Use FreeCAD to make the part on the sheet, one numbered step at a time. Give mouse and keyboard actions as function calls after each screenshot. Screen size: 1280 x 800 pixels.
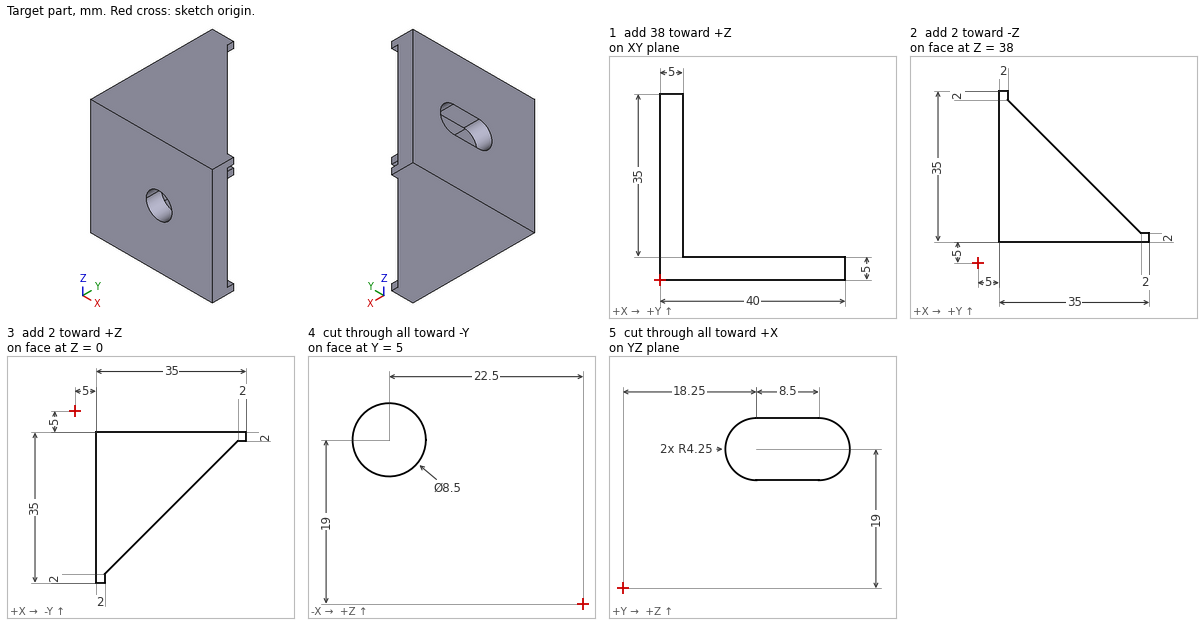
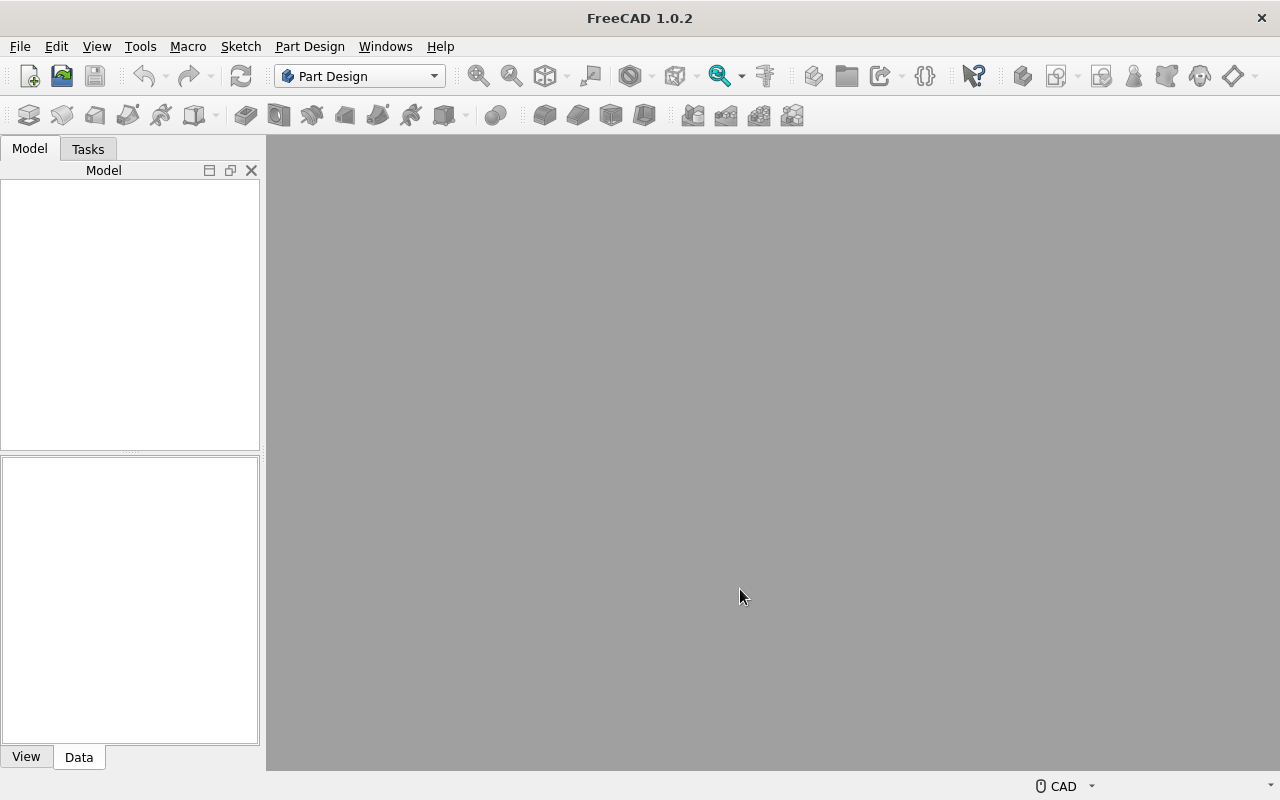
click(29, 76)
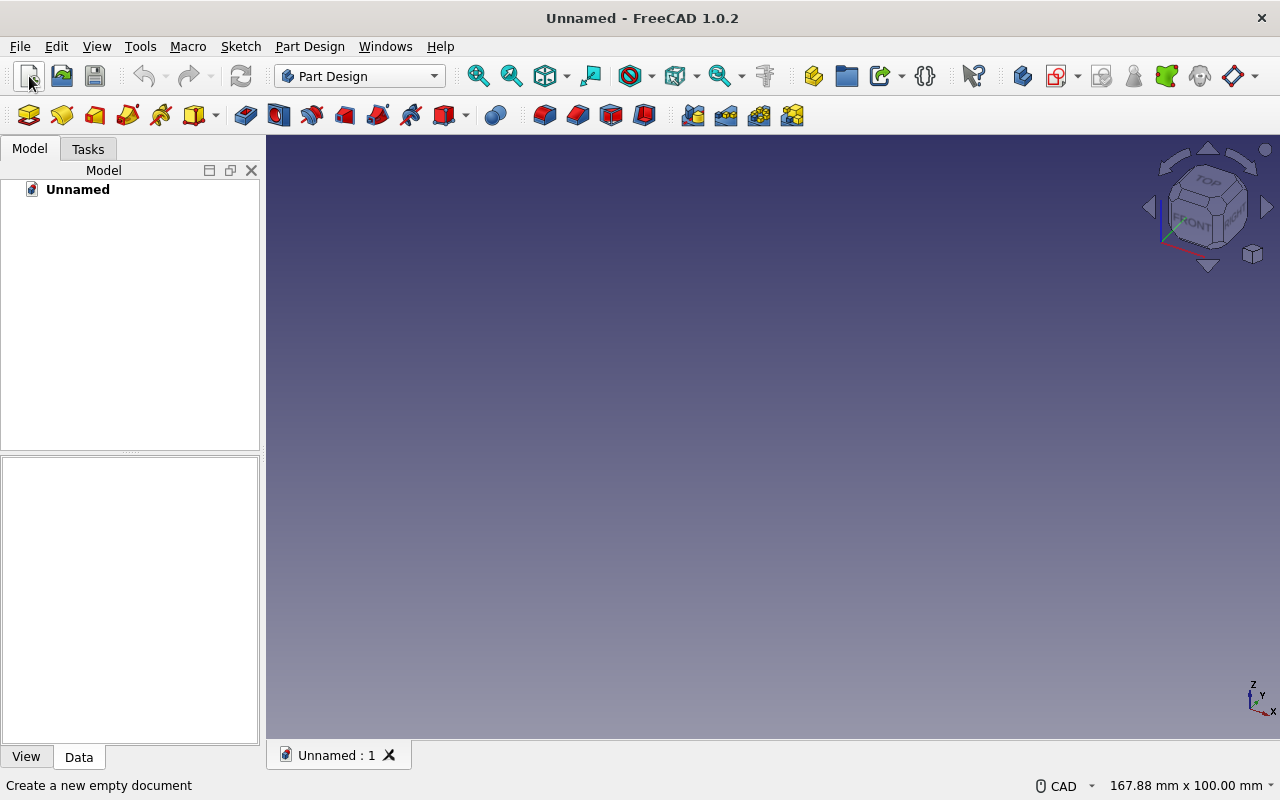
click(1056, 76)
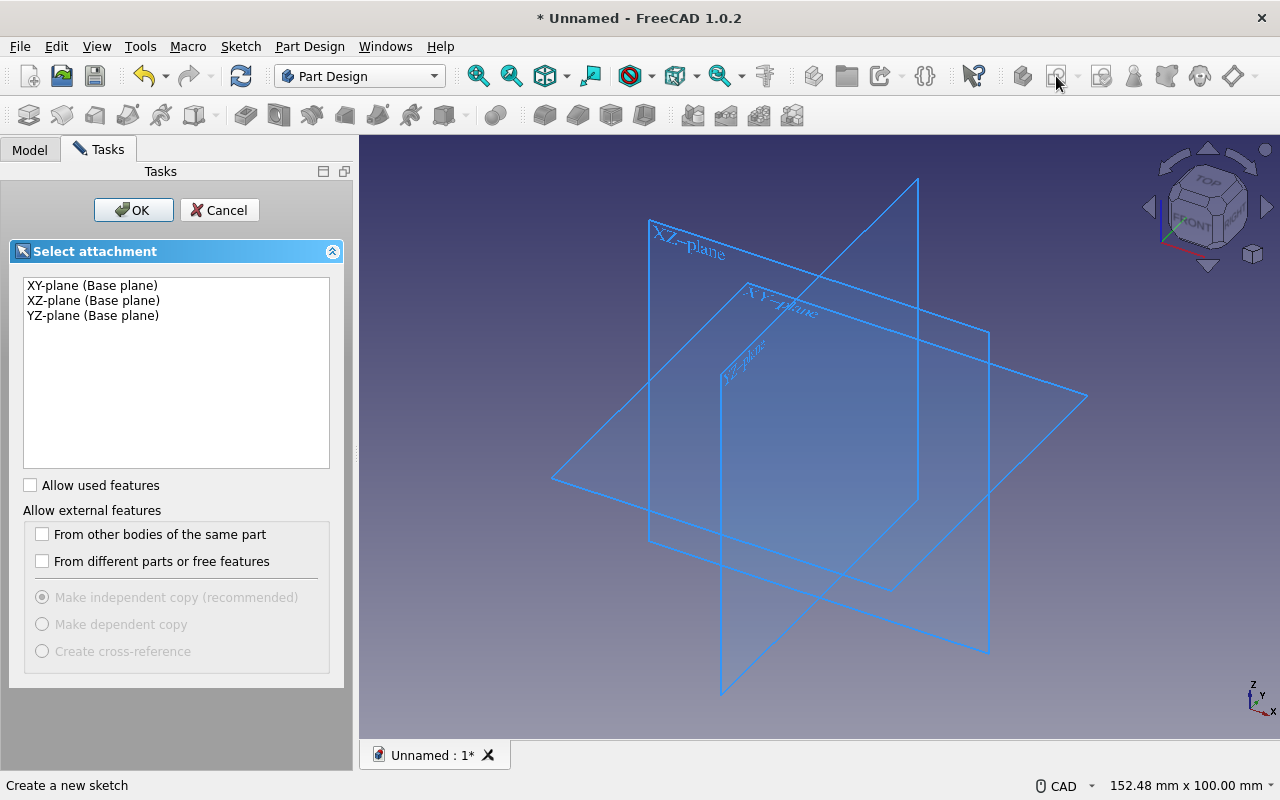
click(84, 286)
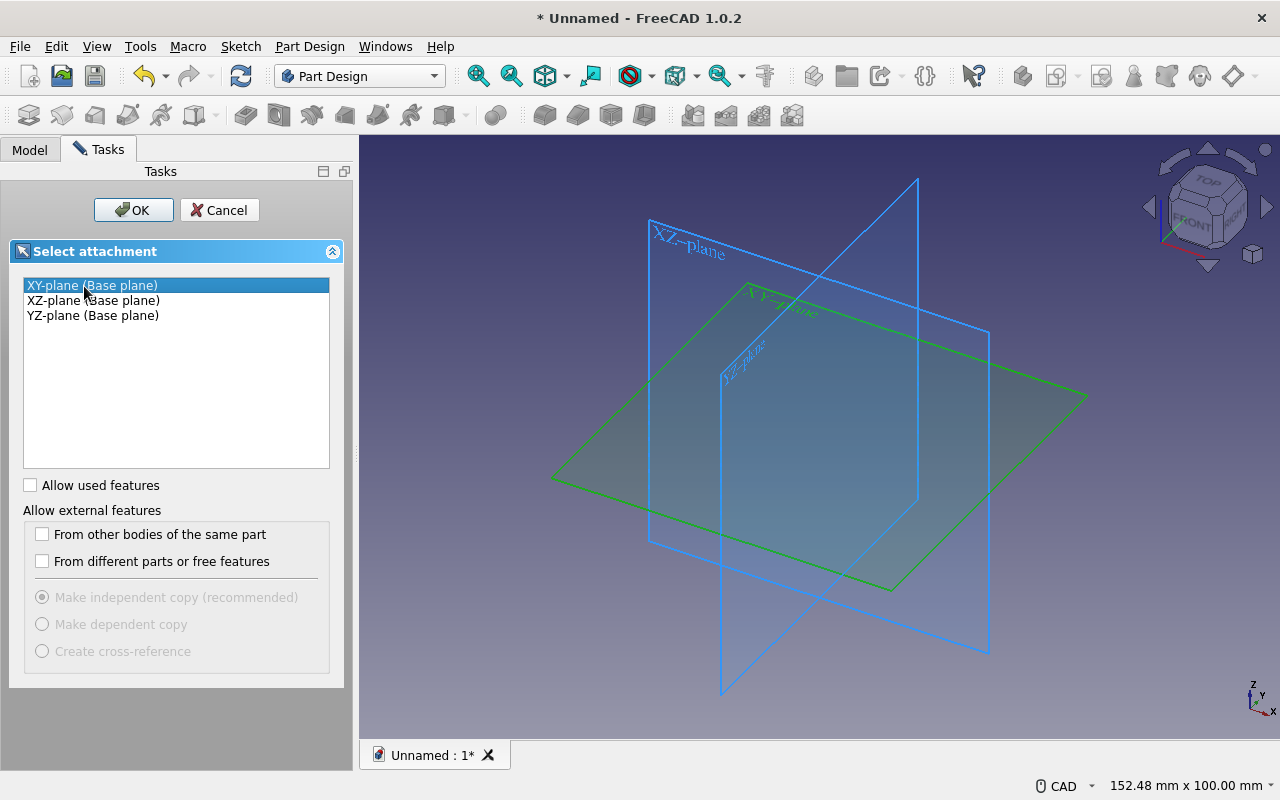
click(134, 210)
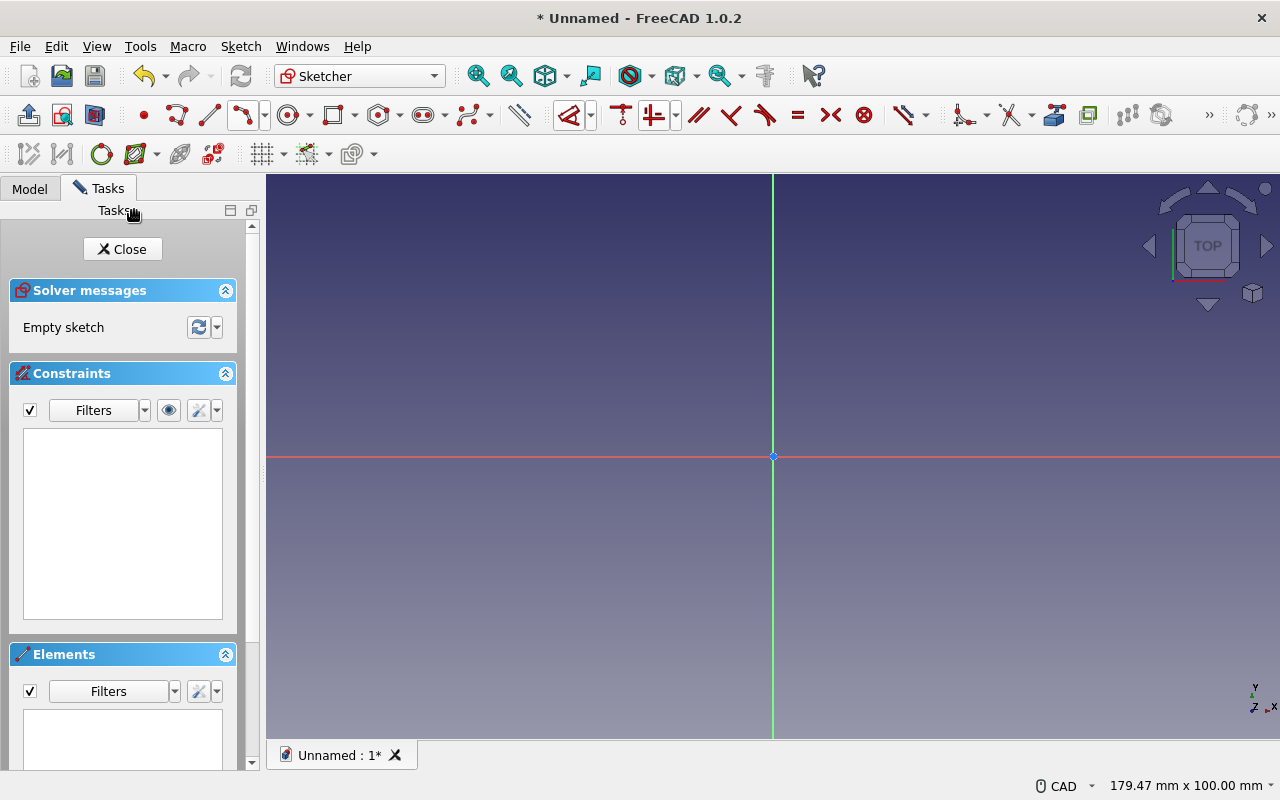
scroll(1115, 202, up, 2)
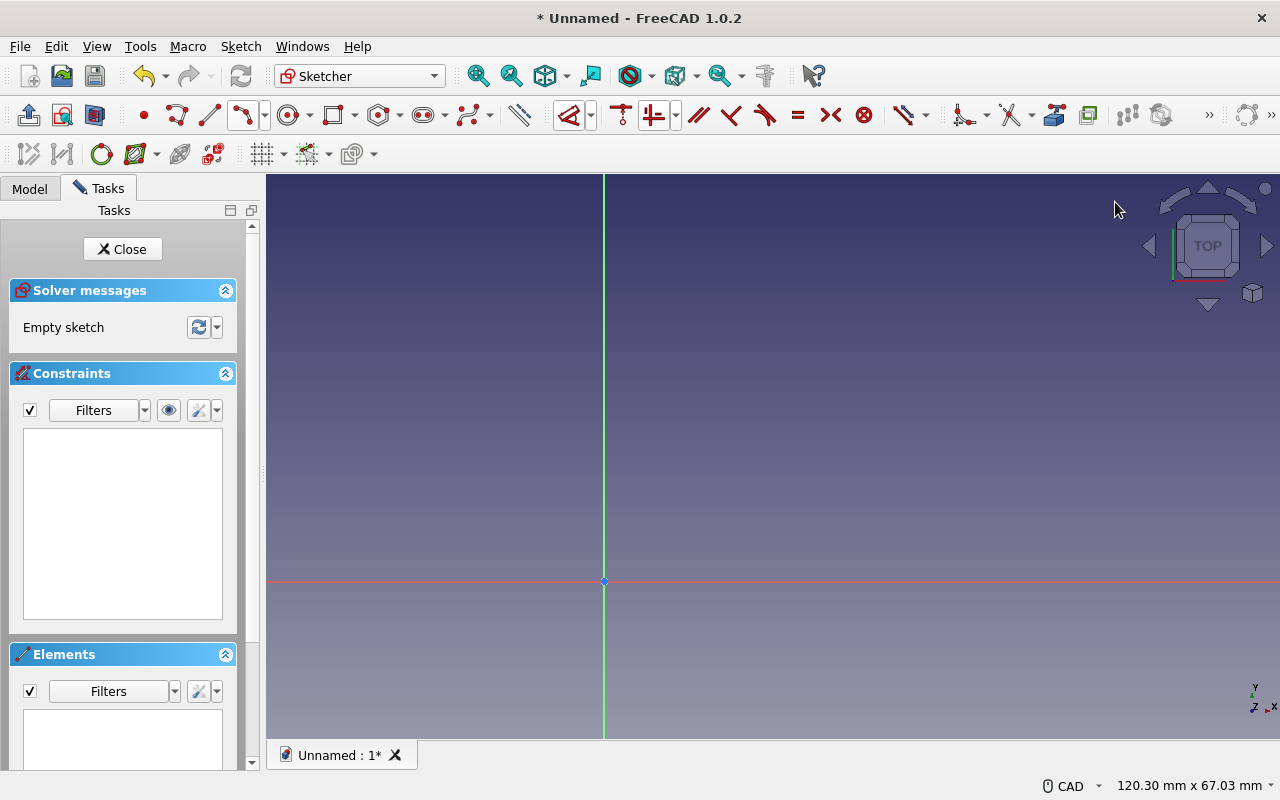
click(177, 116)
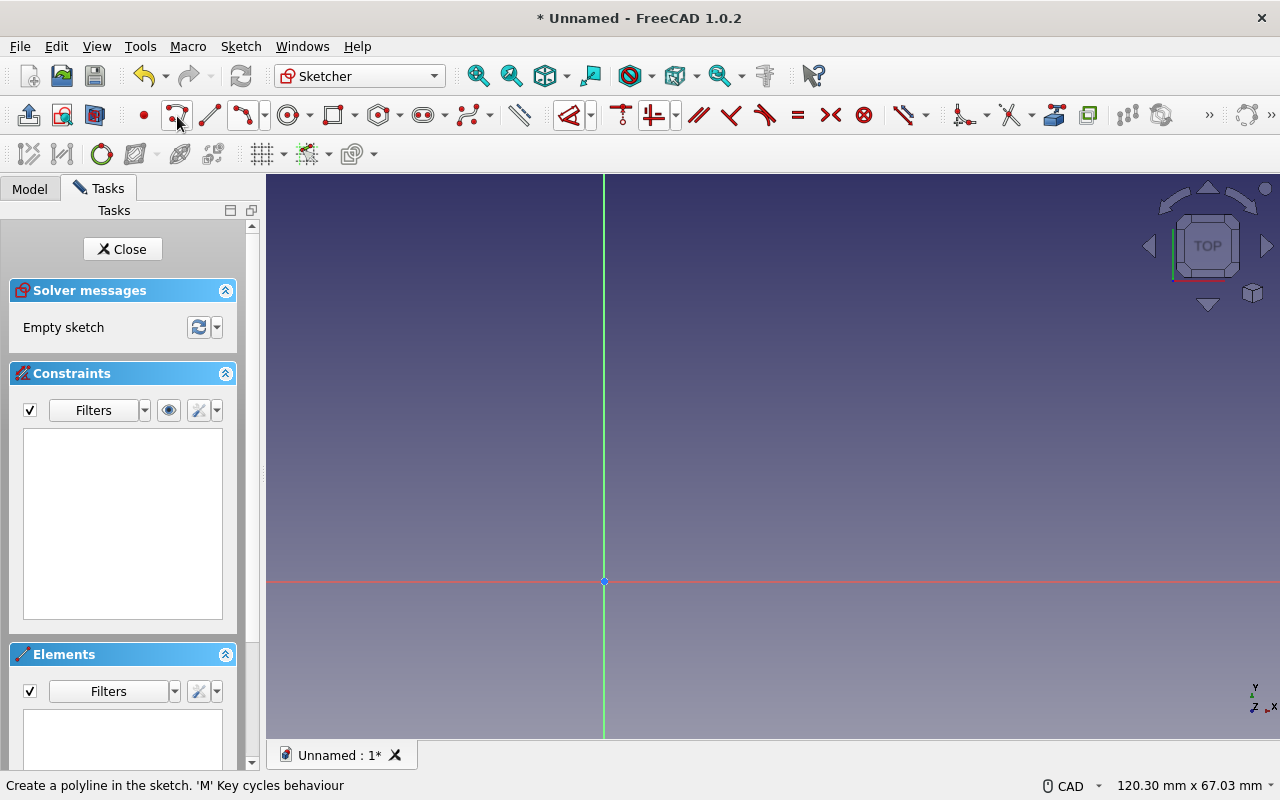
click(604, 582)
click(942, 573)
click(942, 540)
click(647, 540)
click(647, 244)
click(613, 244)
click(604, 582)
key(Escape)
key(Escape)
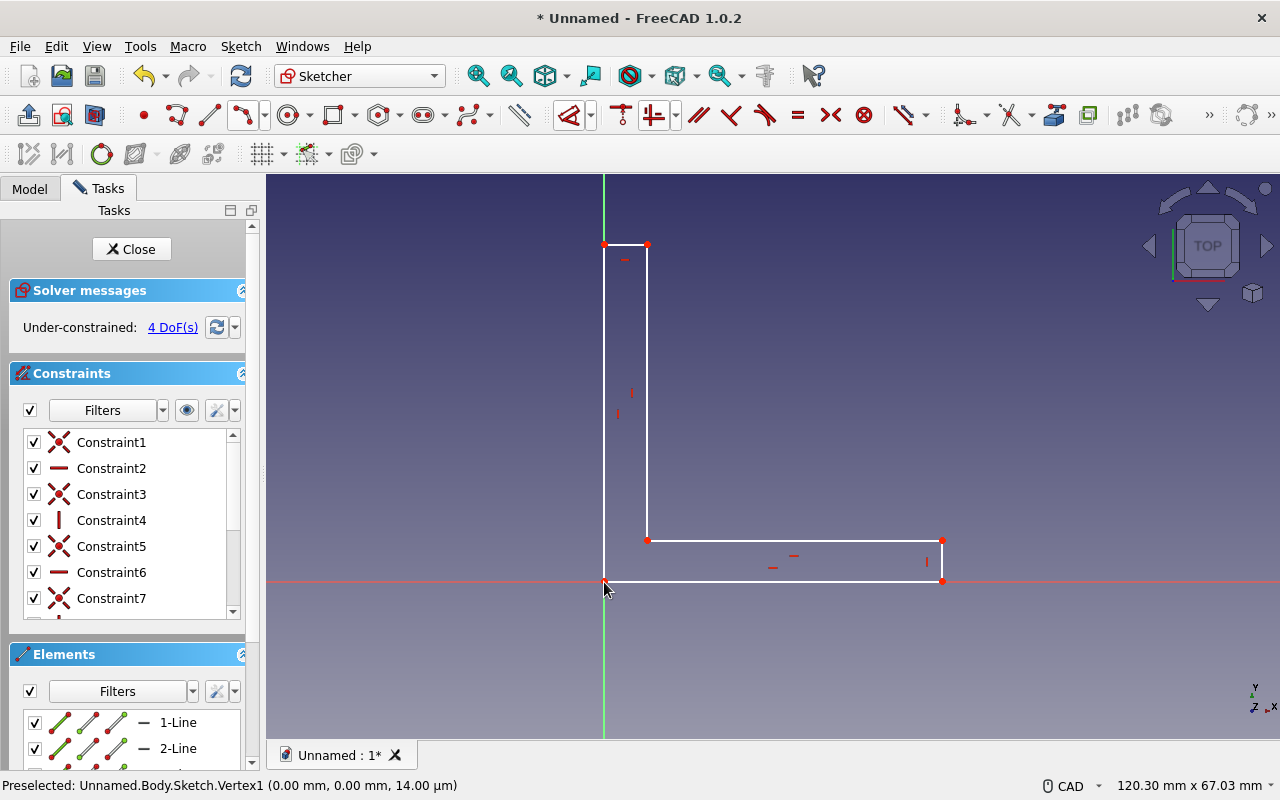
click(942, 569)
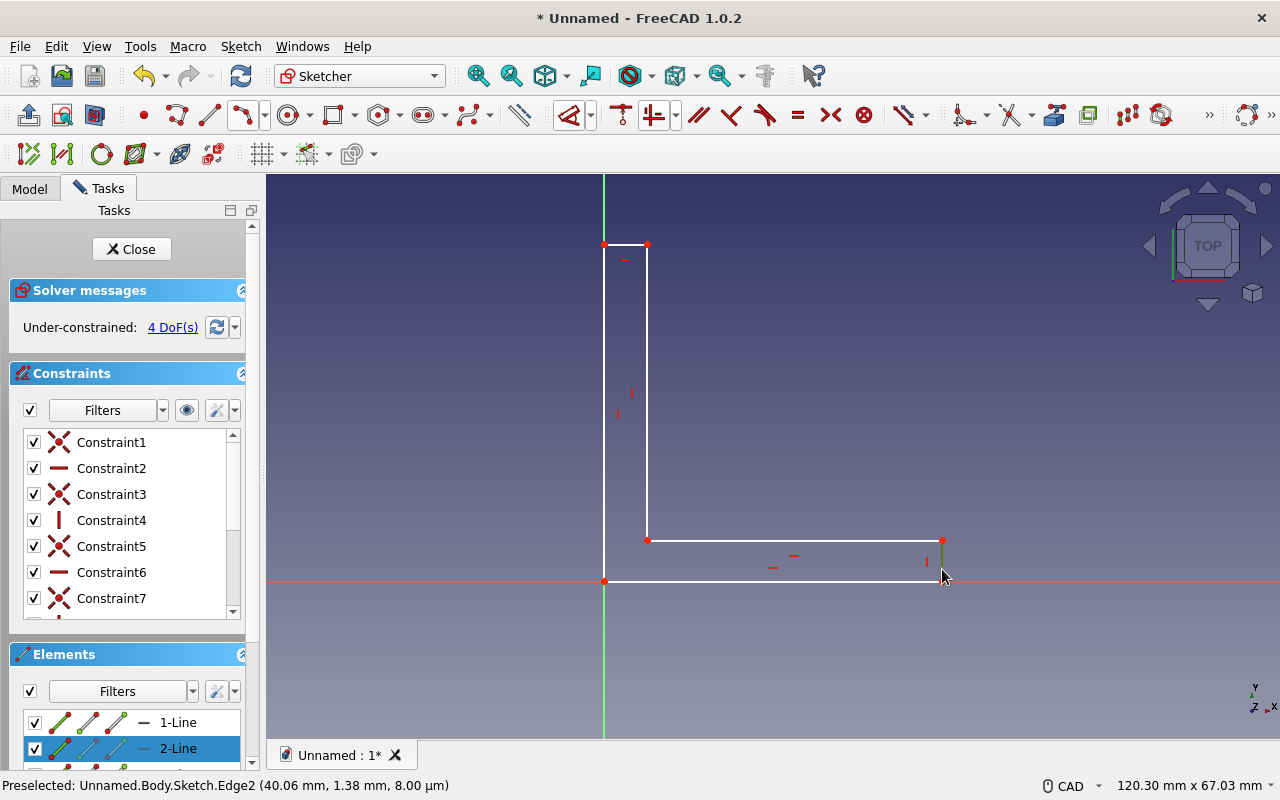
key(i)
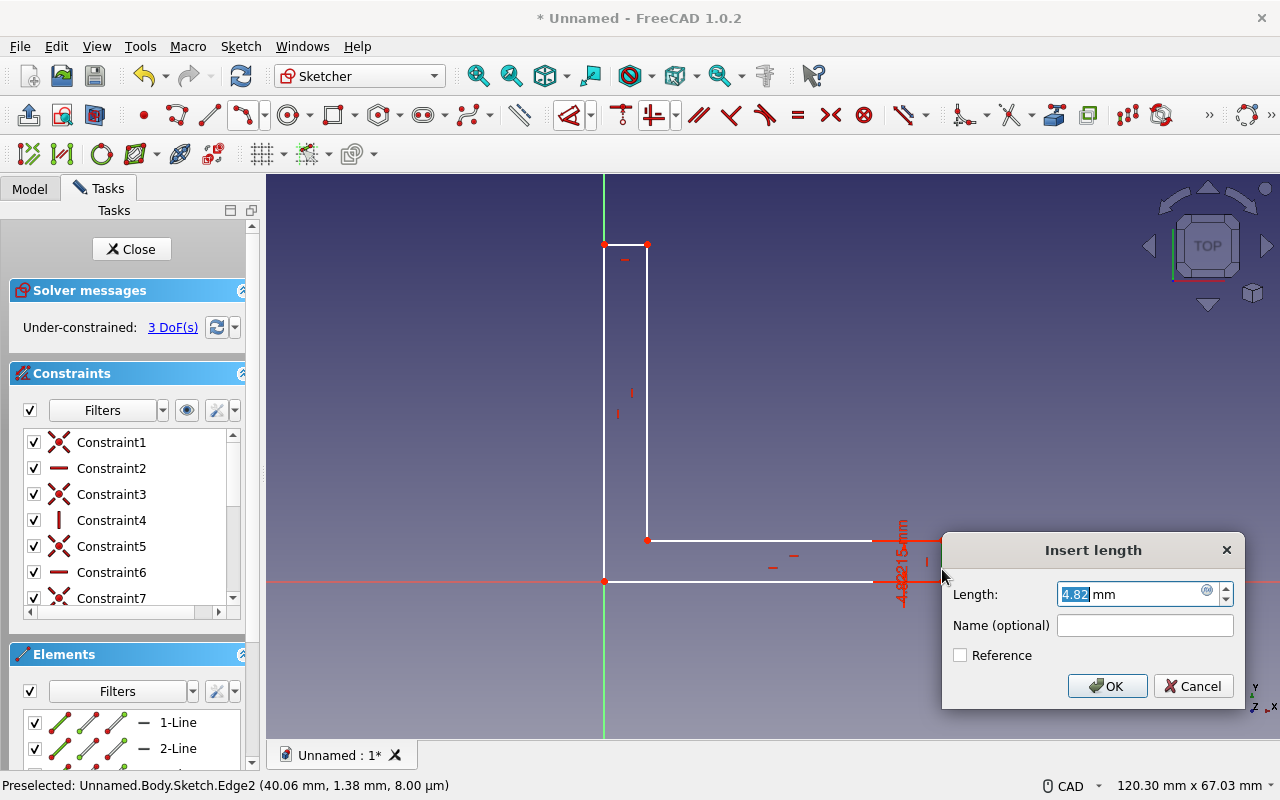
text(5)
key(Return)